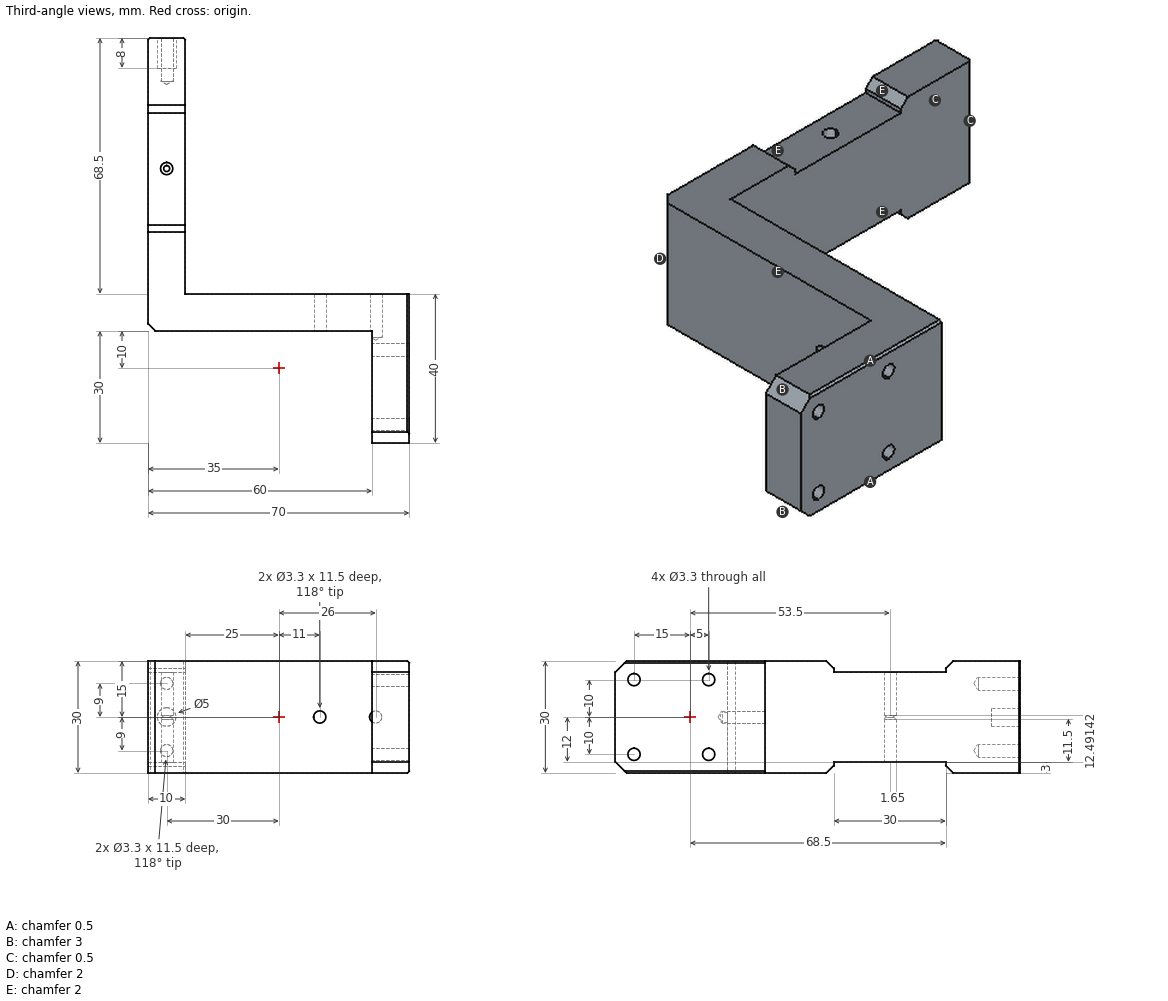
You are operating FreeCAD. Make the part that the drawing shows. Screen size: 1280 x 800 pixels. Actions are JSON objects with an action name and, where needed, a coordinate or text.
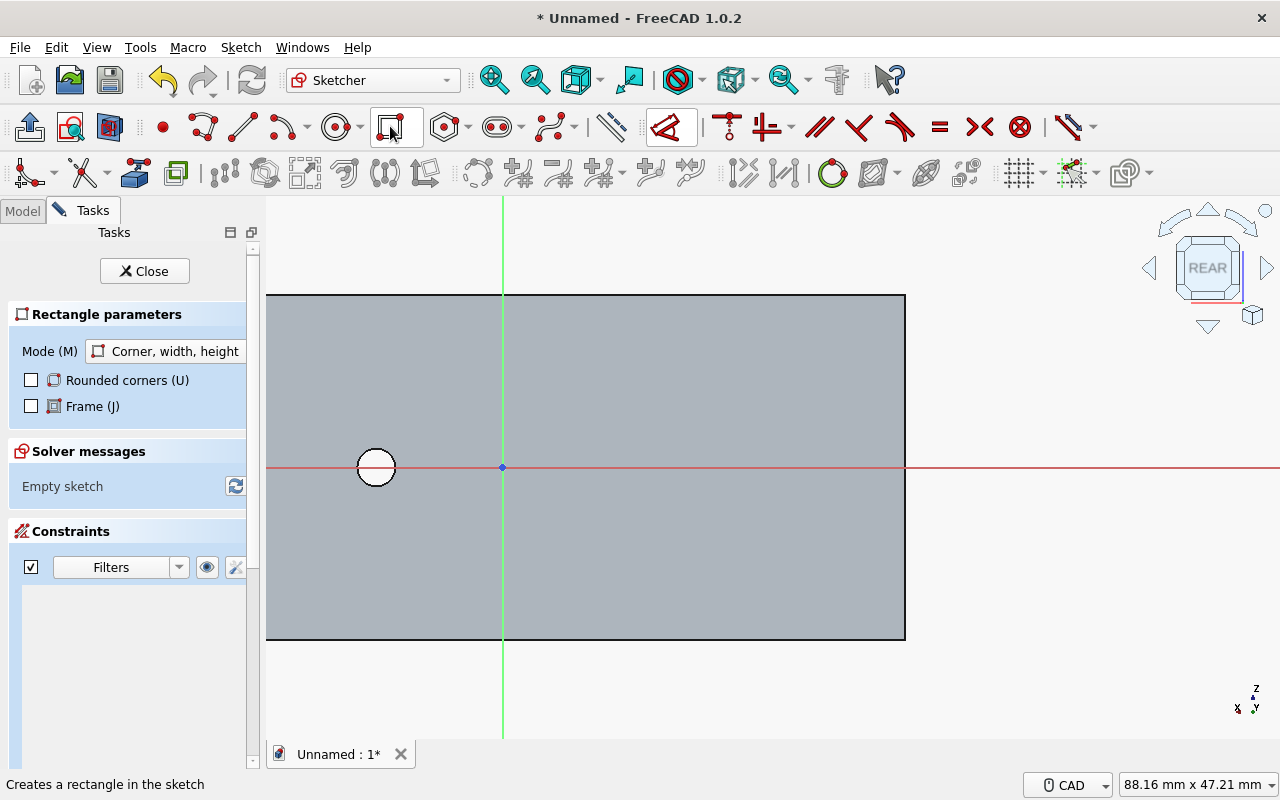
{"action": "left_click", "coordinate": [790, 295]}
{"action": "left_click", "coordinate": [905, 640]}
{"action": "key", "text": "Escape"}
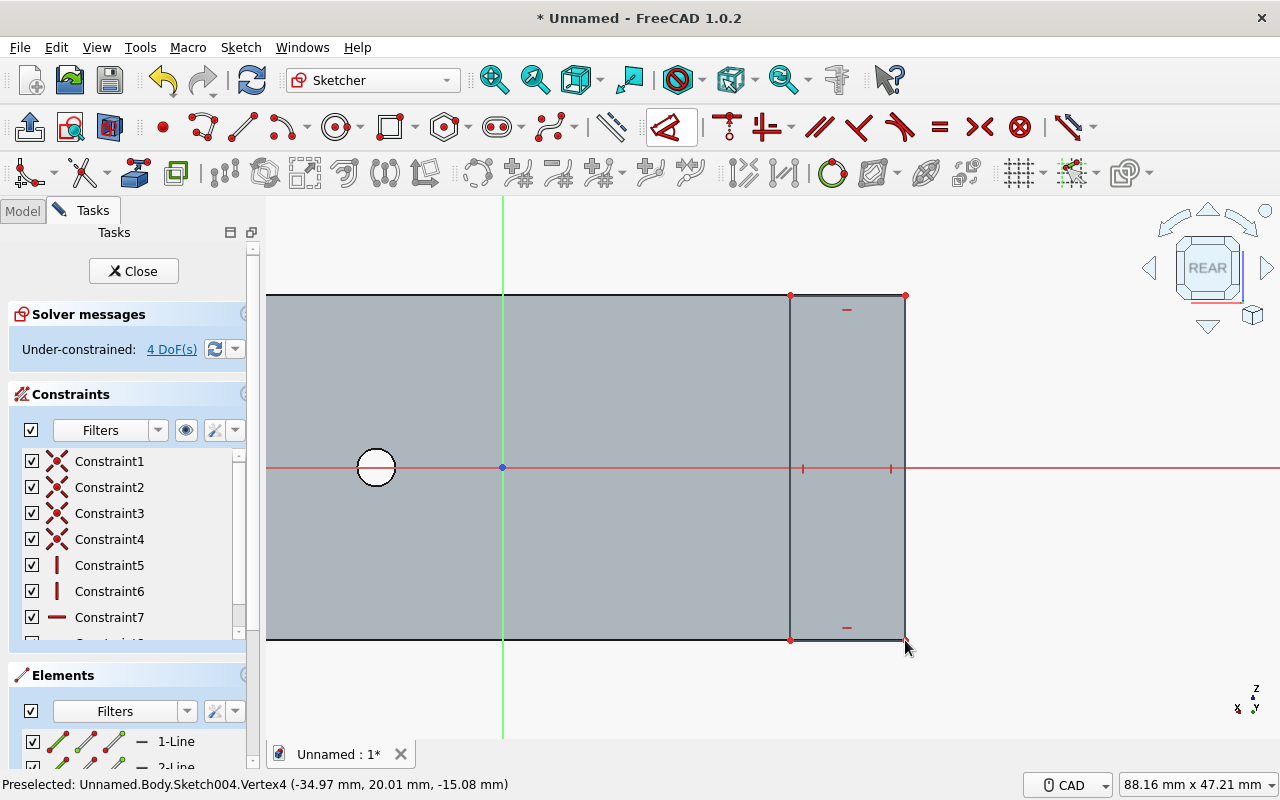
{"action": "left_click", "coordinate": [790, 400]}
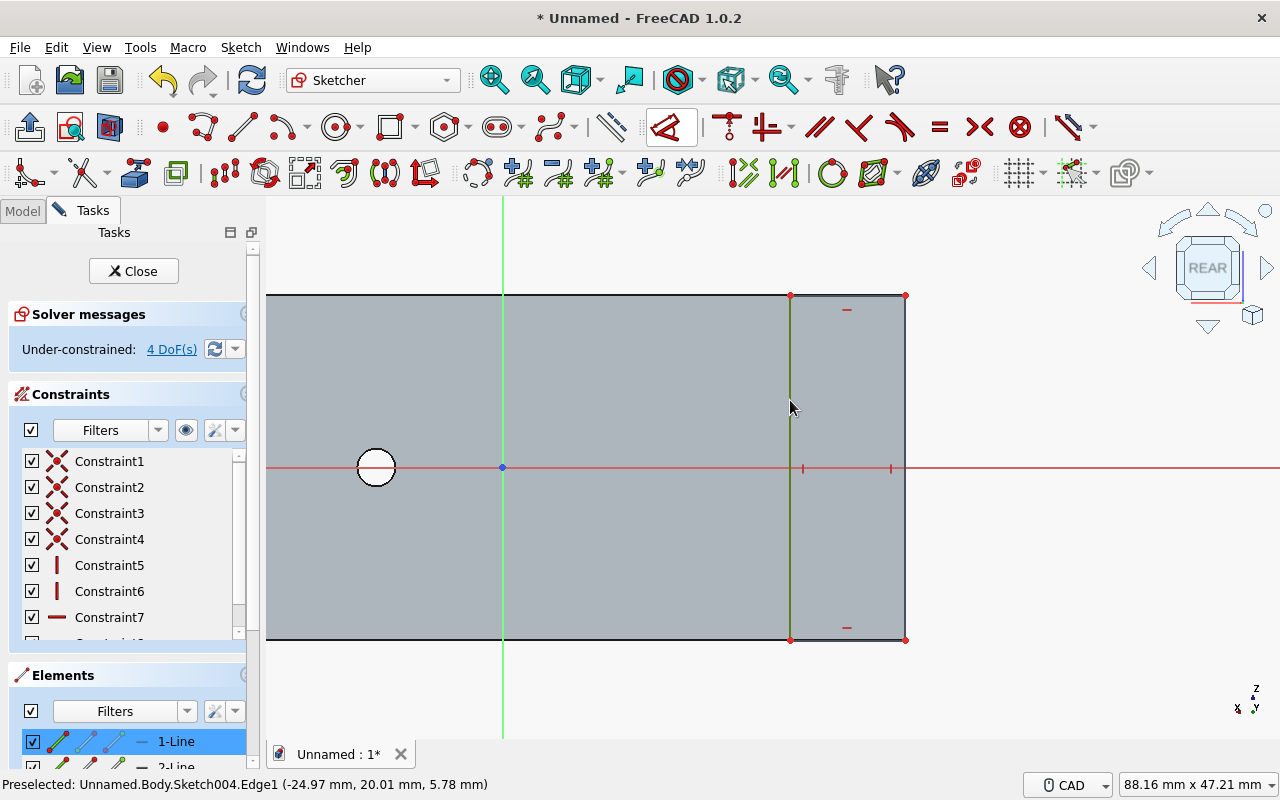
{"action": "key", "text": "i"}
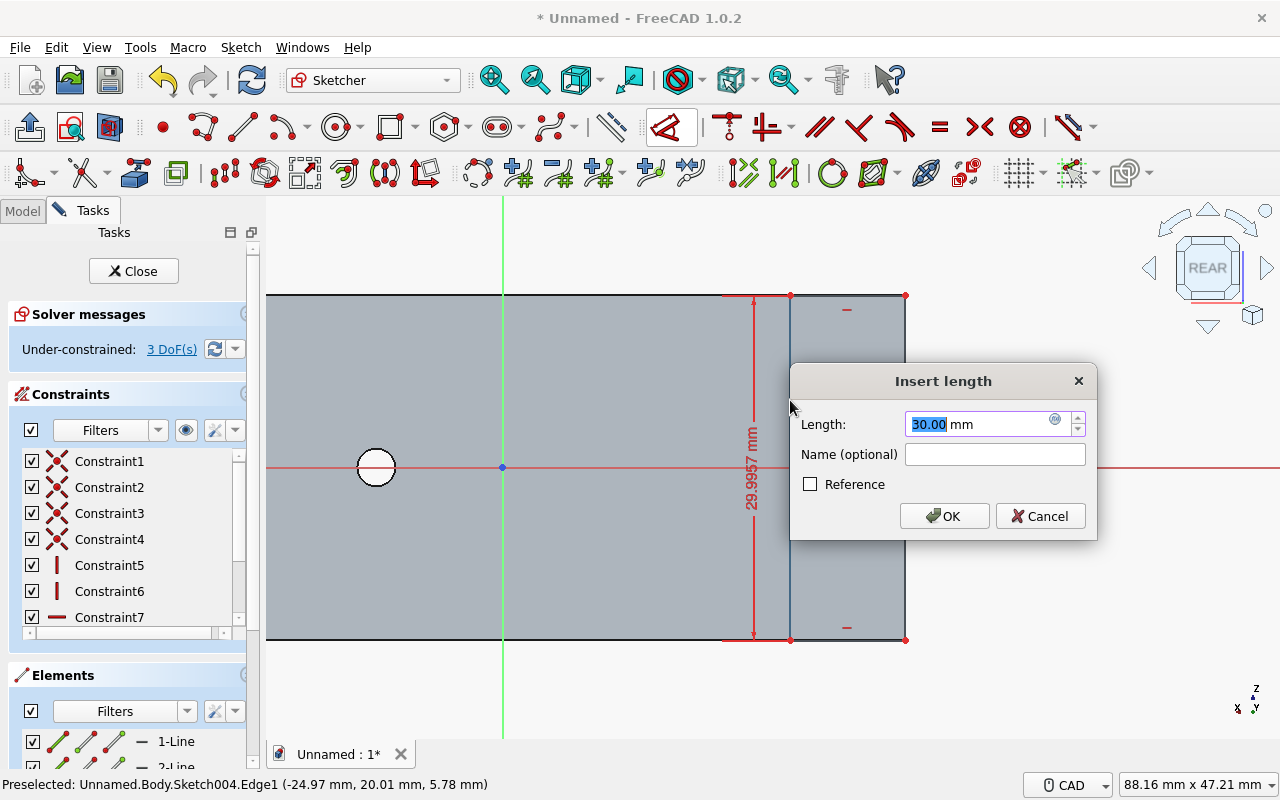
{"action": "type", "text": "30"}
{"action": "key", "text": "Return"}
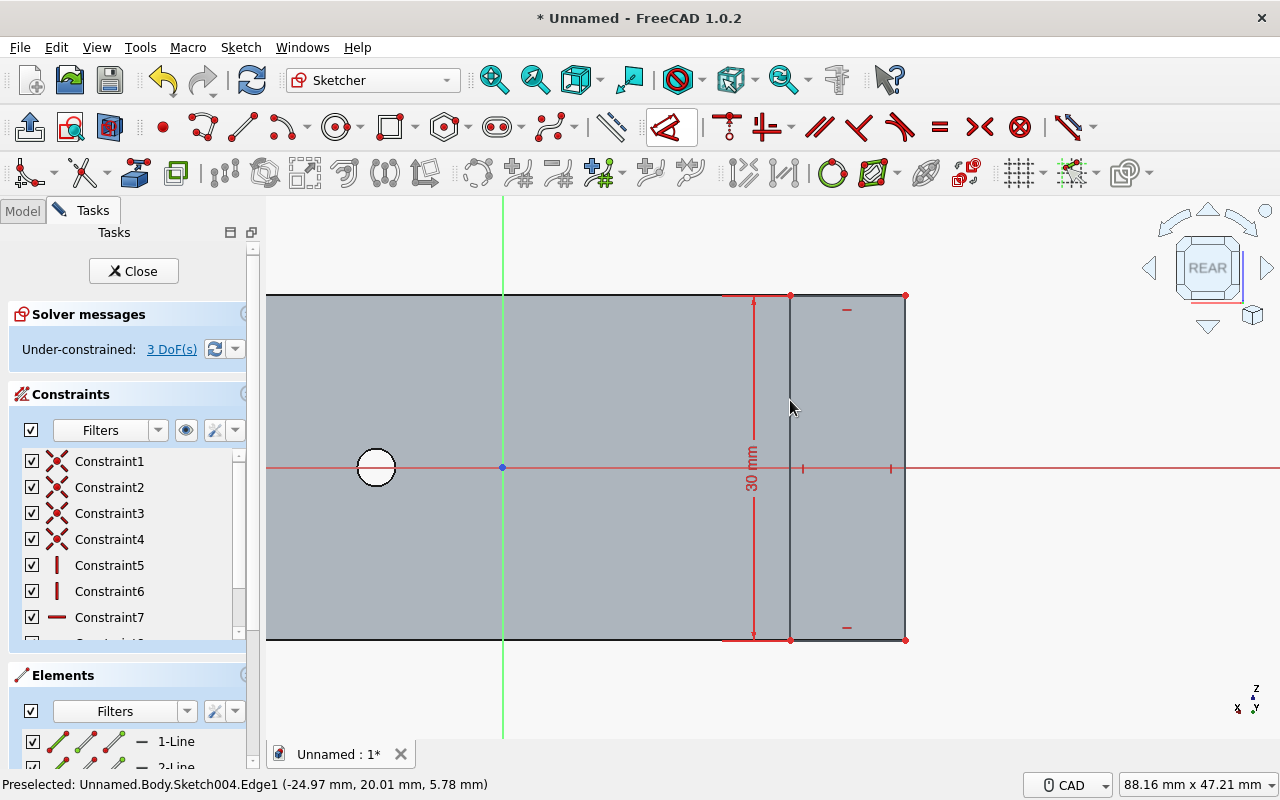
{"action": "left_click", "coordinate": [824, 641]}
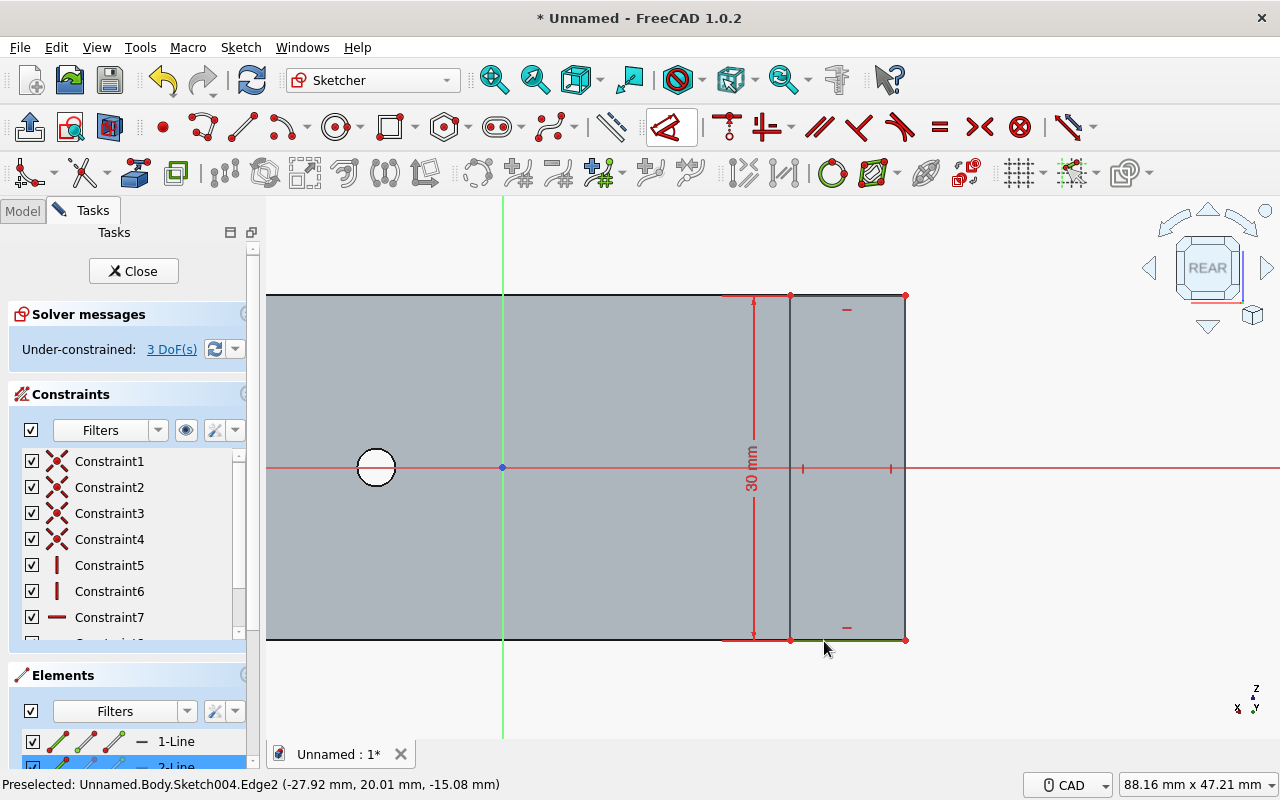
{"action": "key", "text": "l"}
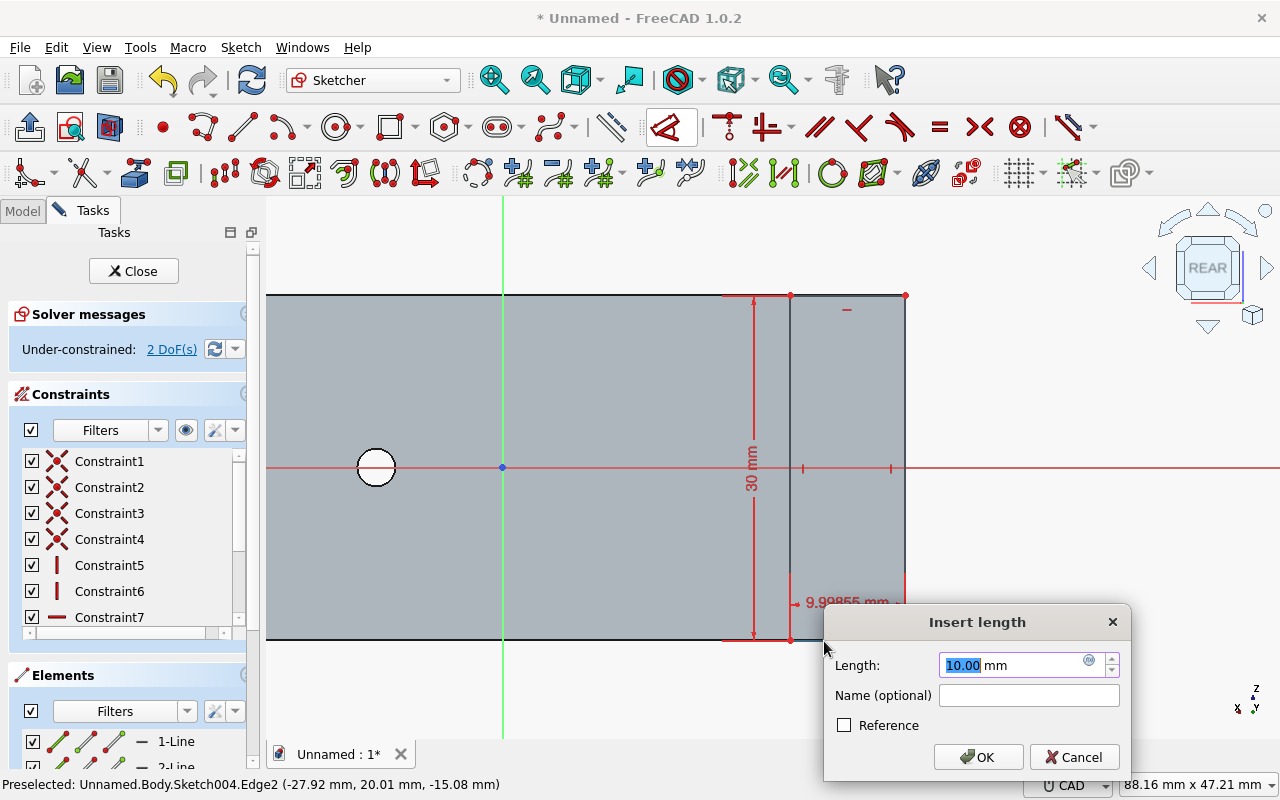
{"action": "type", "text": "10"}
{"action": "key", "text": "Return"}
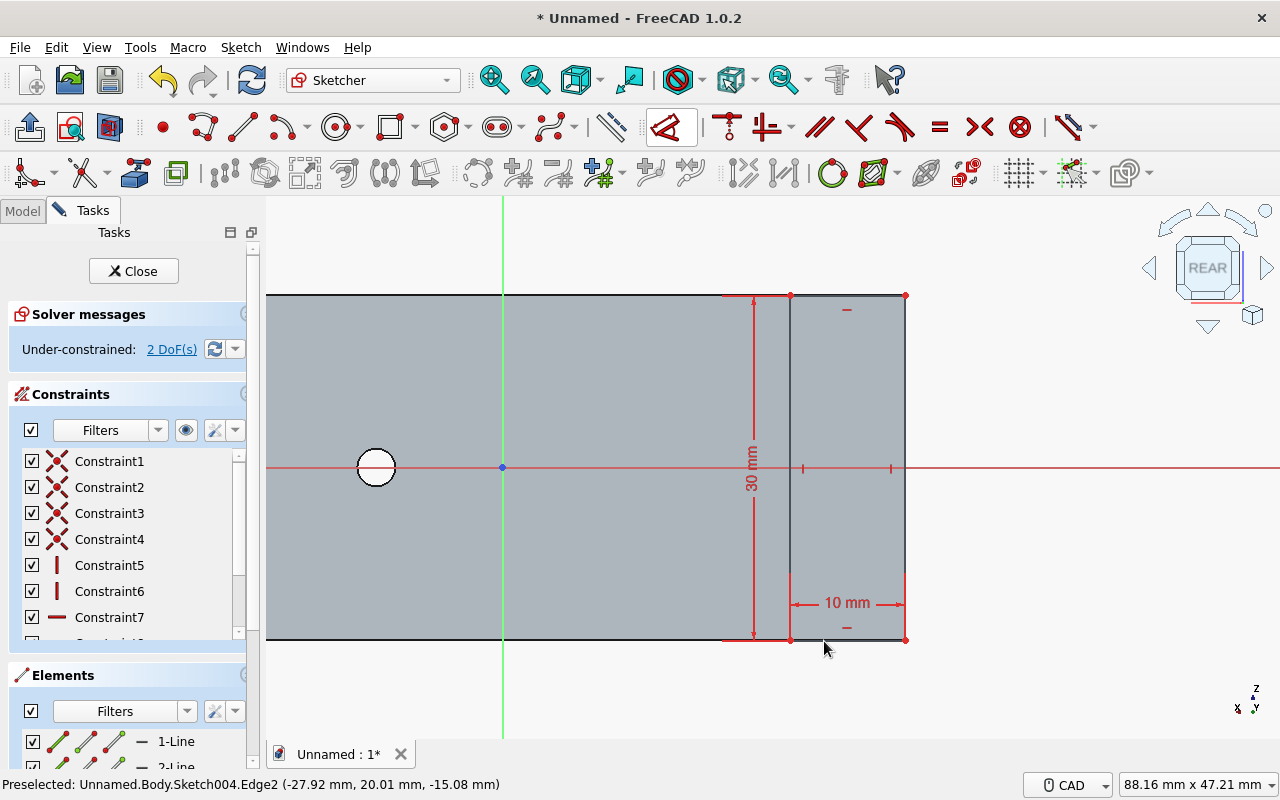
{"action": "left_click", "coordinate": [790, 296]}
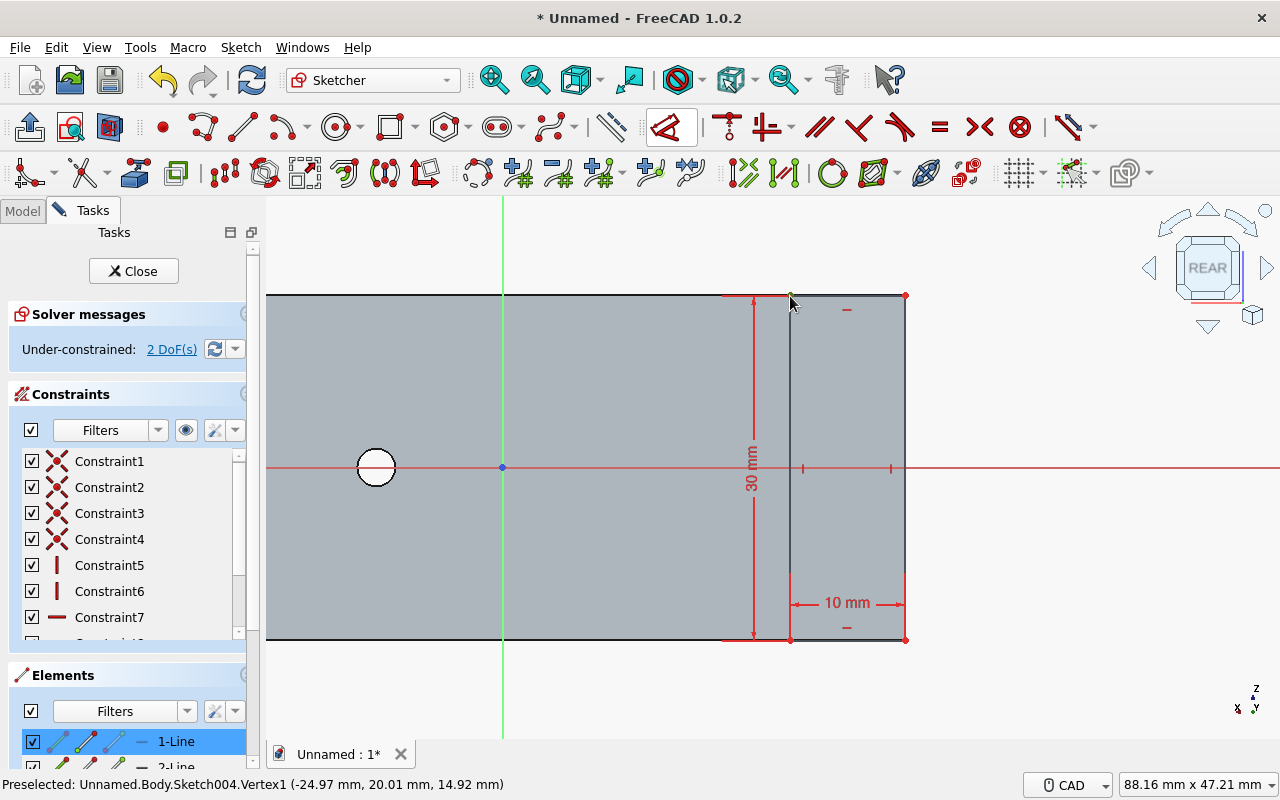
{"action": "key", "text": "l"}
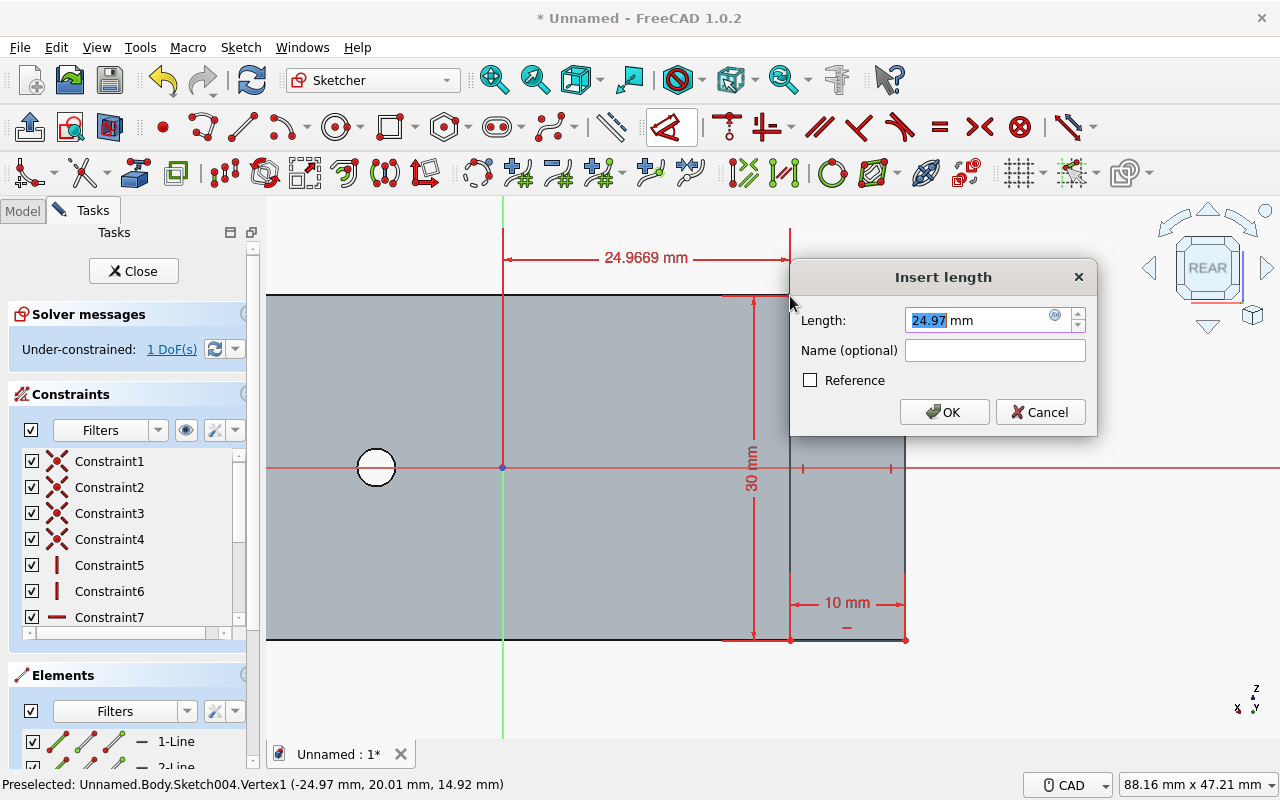
{"action": "type", "text": "25"}
{"action": "key", "text": "Return"}